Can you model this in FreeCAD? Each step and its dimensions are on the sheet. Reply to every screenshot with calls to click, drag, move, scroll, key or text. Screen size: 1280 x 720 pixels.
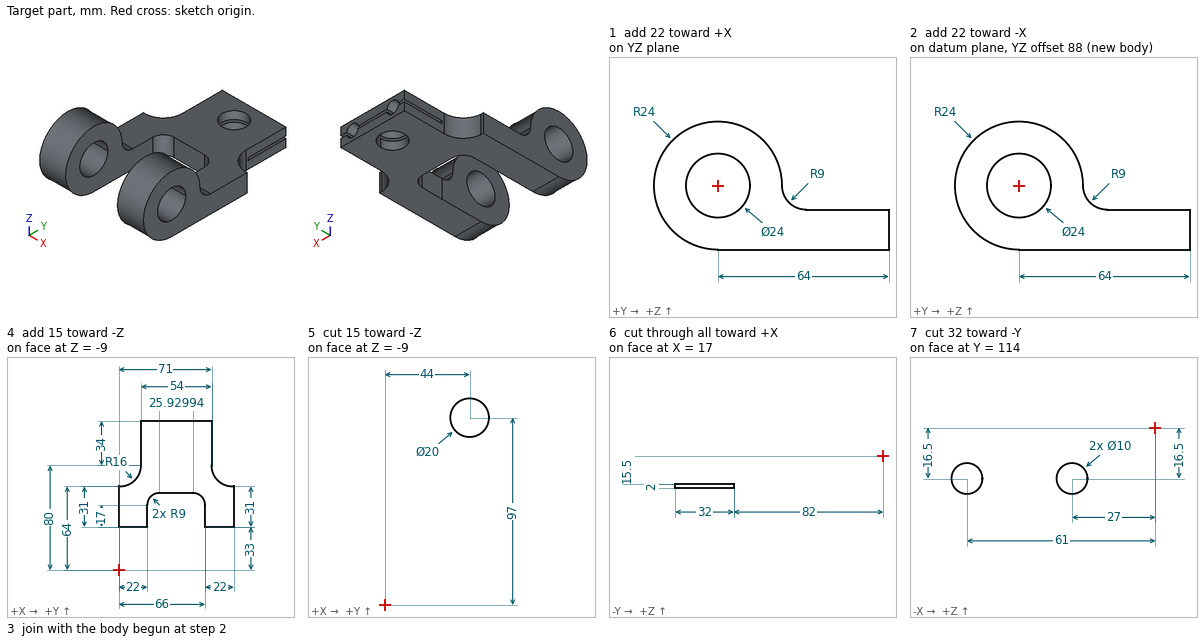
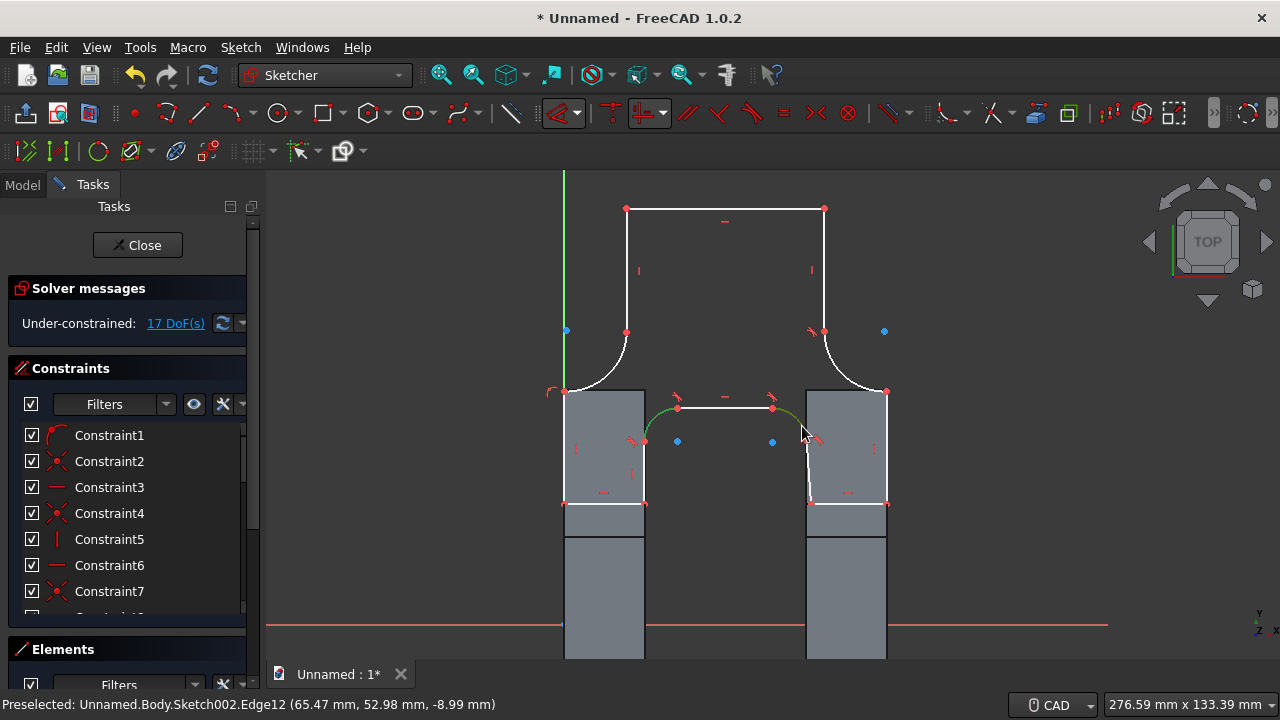
click(784, 114)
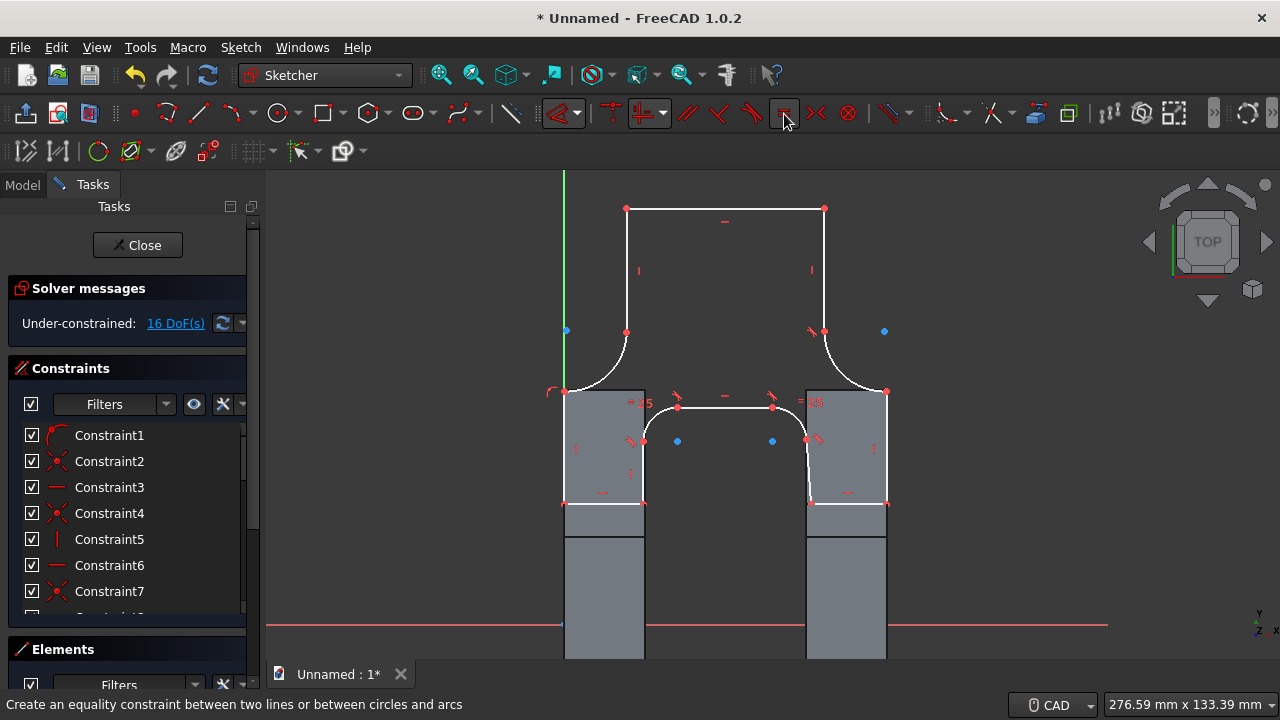
click(662, 411)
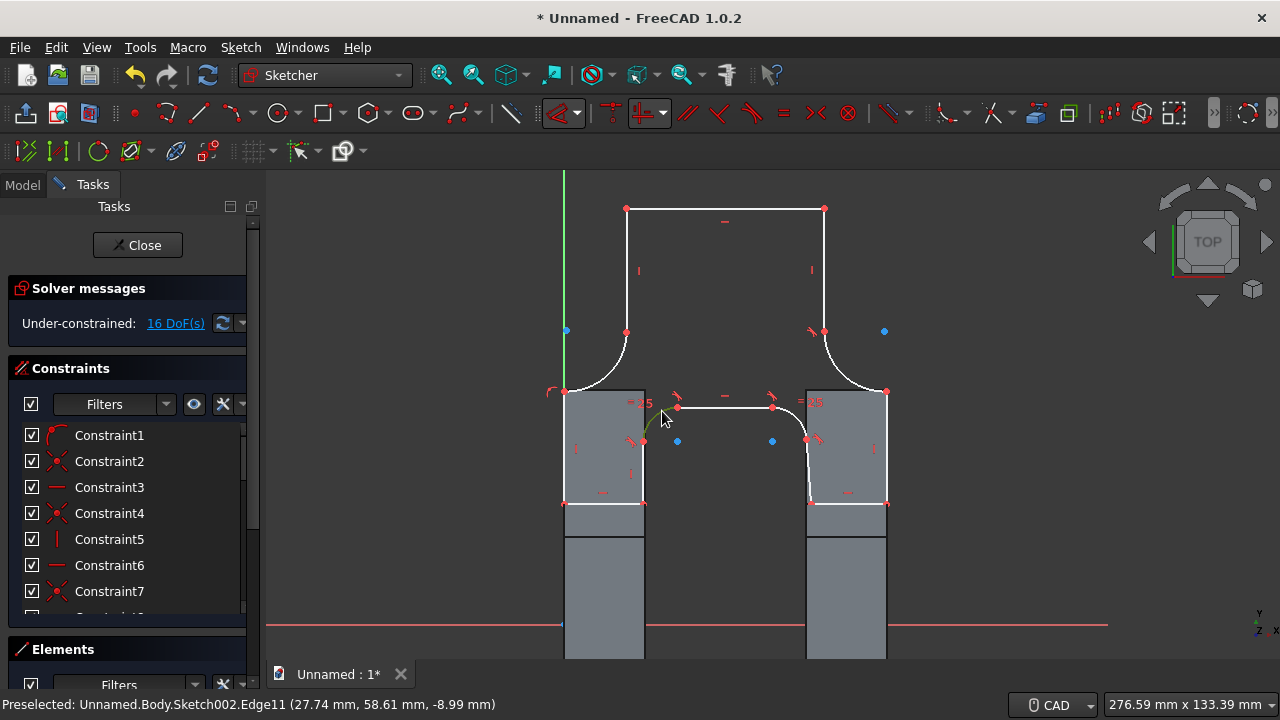
click(580, 114)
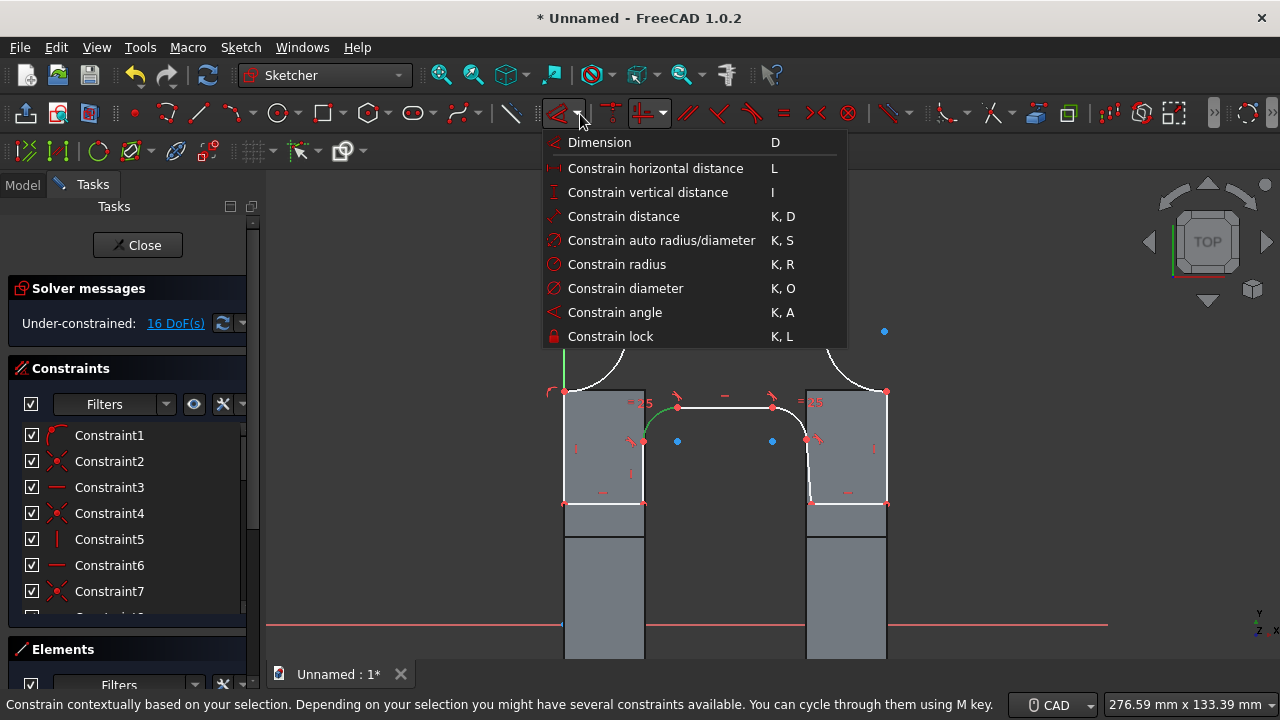
click(695, 264)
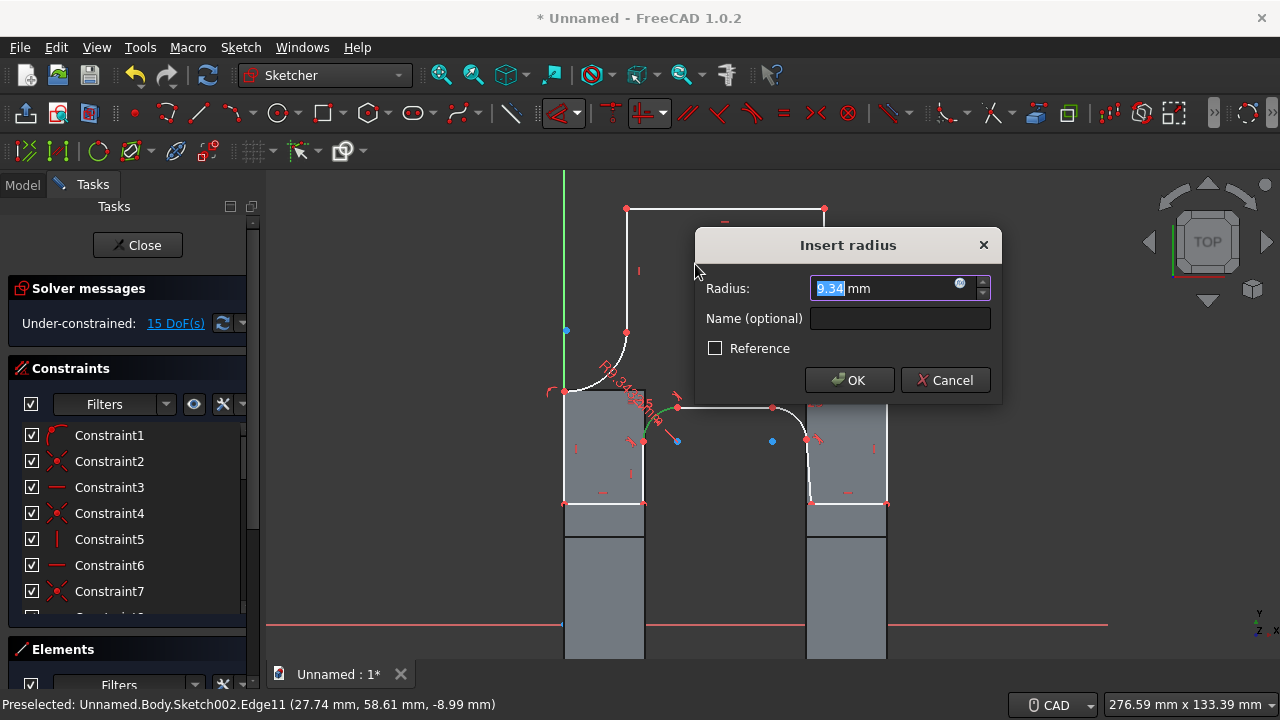
text(9)
key(Return)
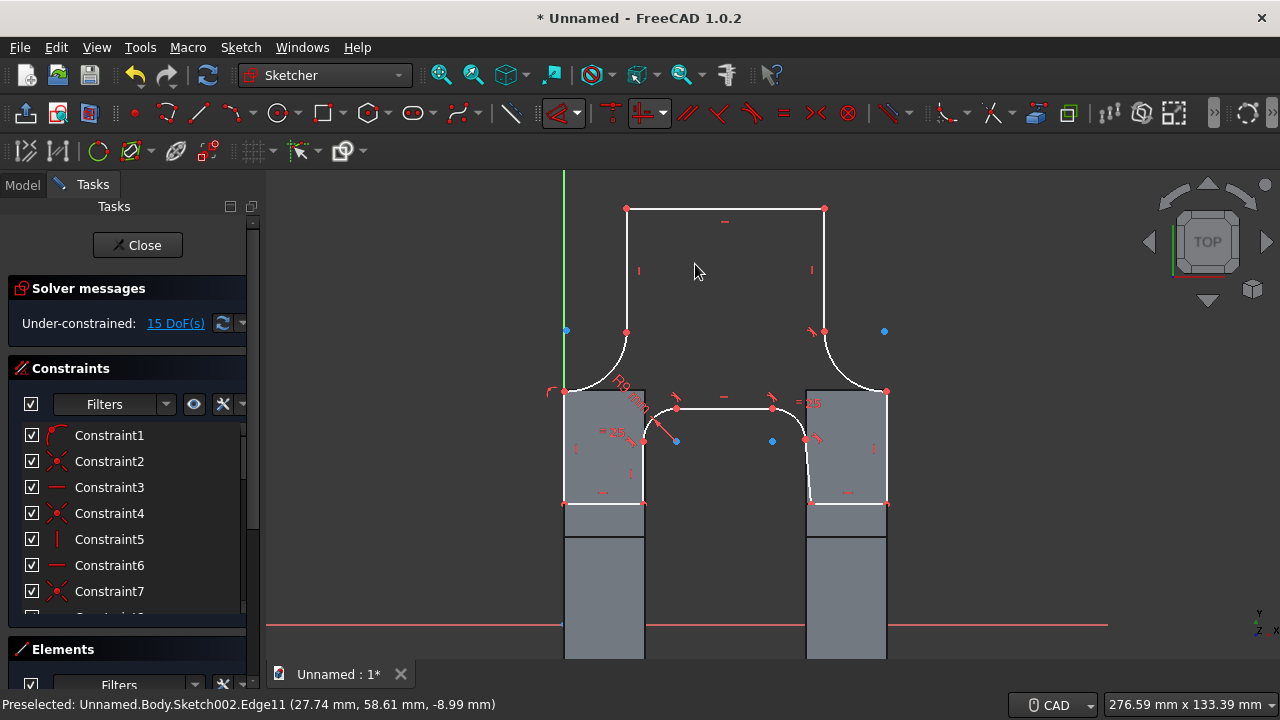
click(831, 359)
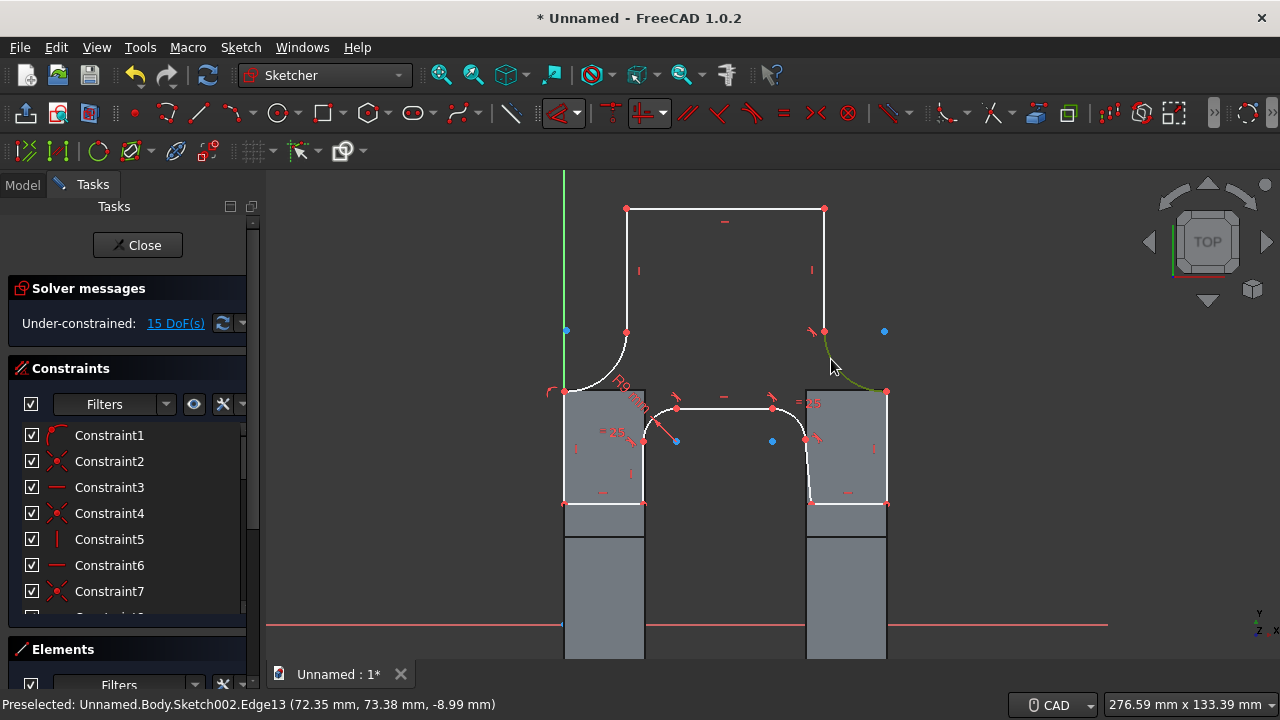
key(k)
key(r)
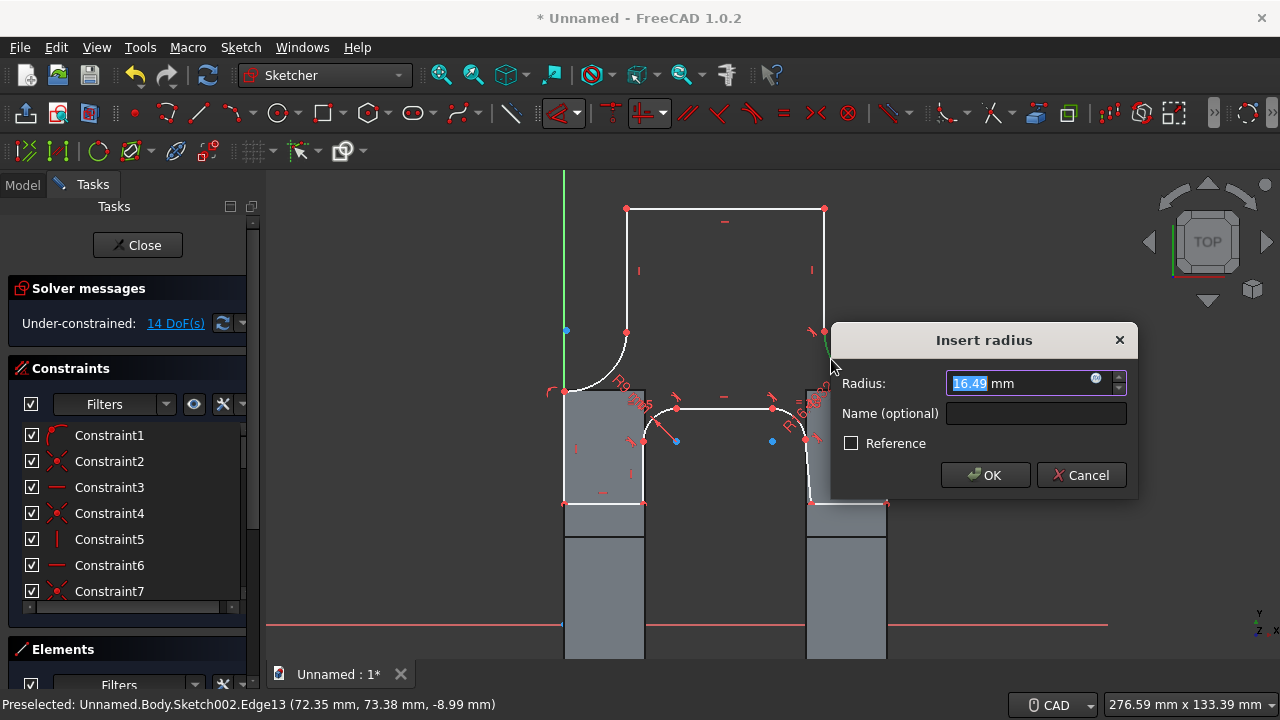
text(16)
key(Return)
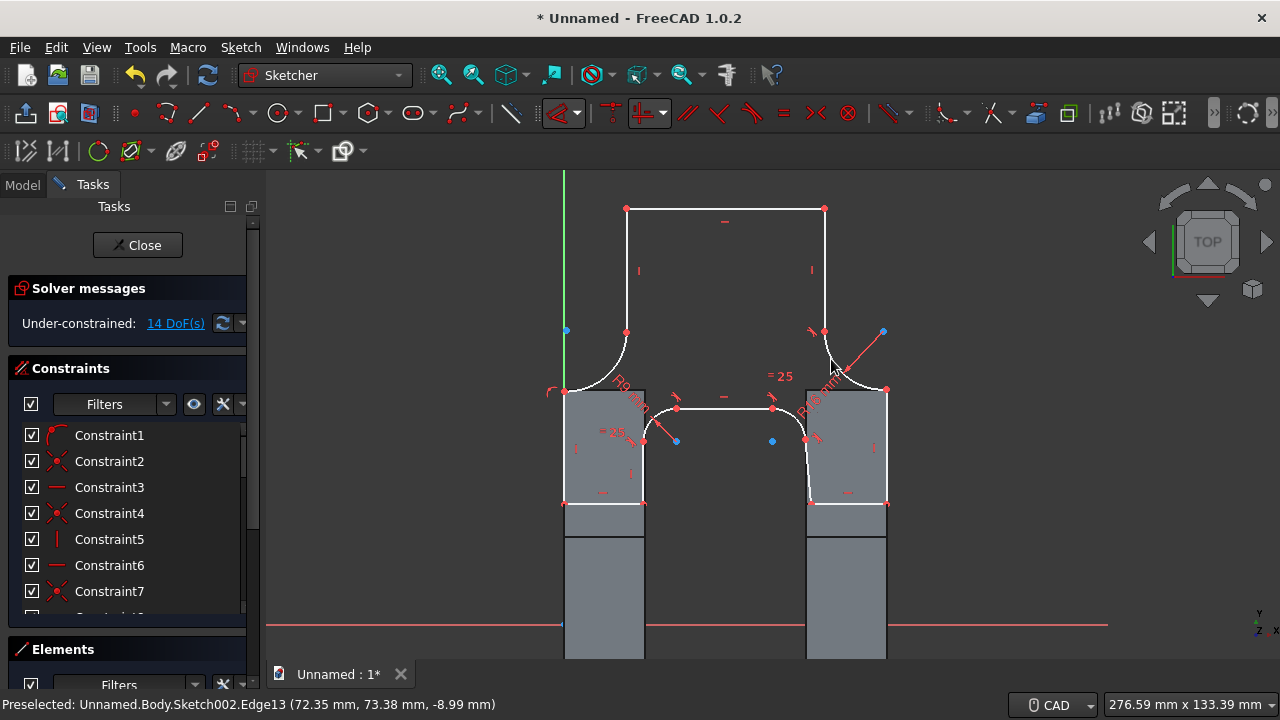
click(592, 386)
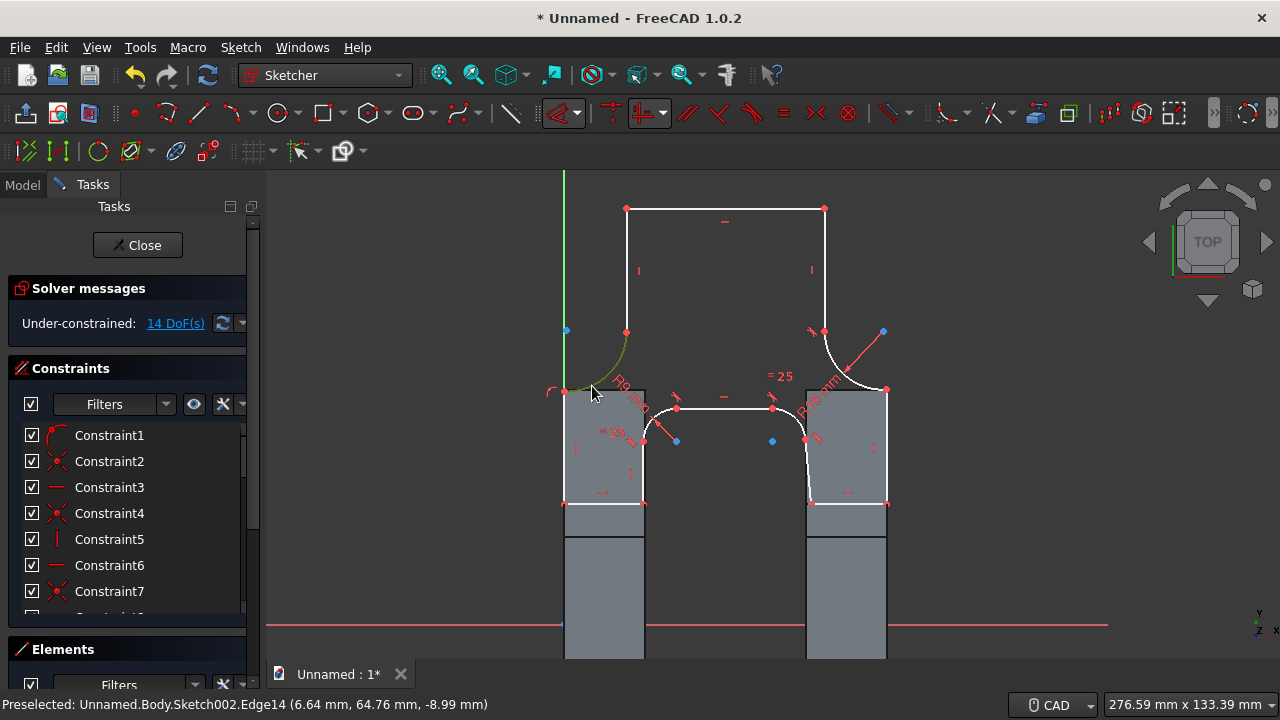
key(k)
key(r)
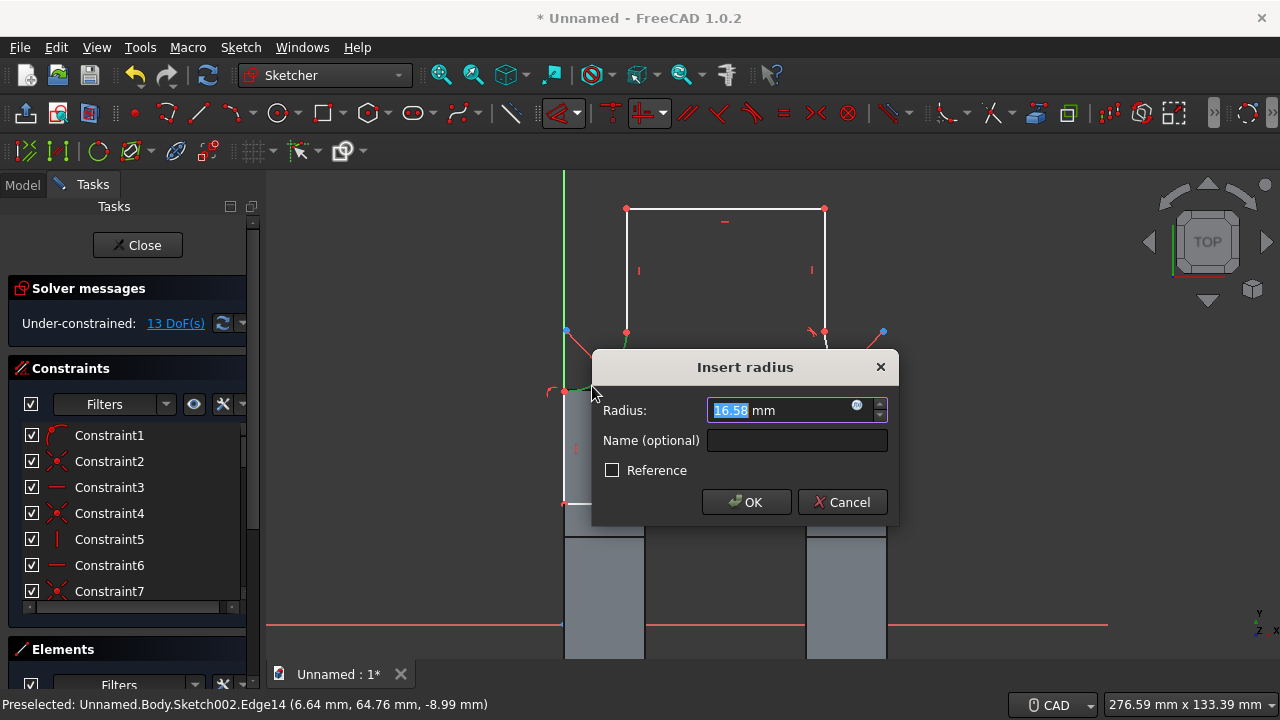
text(16)
key(Return)